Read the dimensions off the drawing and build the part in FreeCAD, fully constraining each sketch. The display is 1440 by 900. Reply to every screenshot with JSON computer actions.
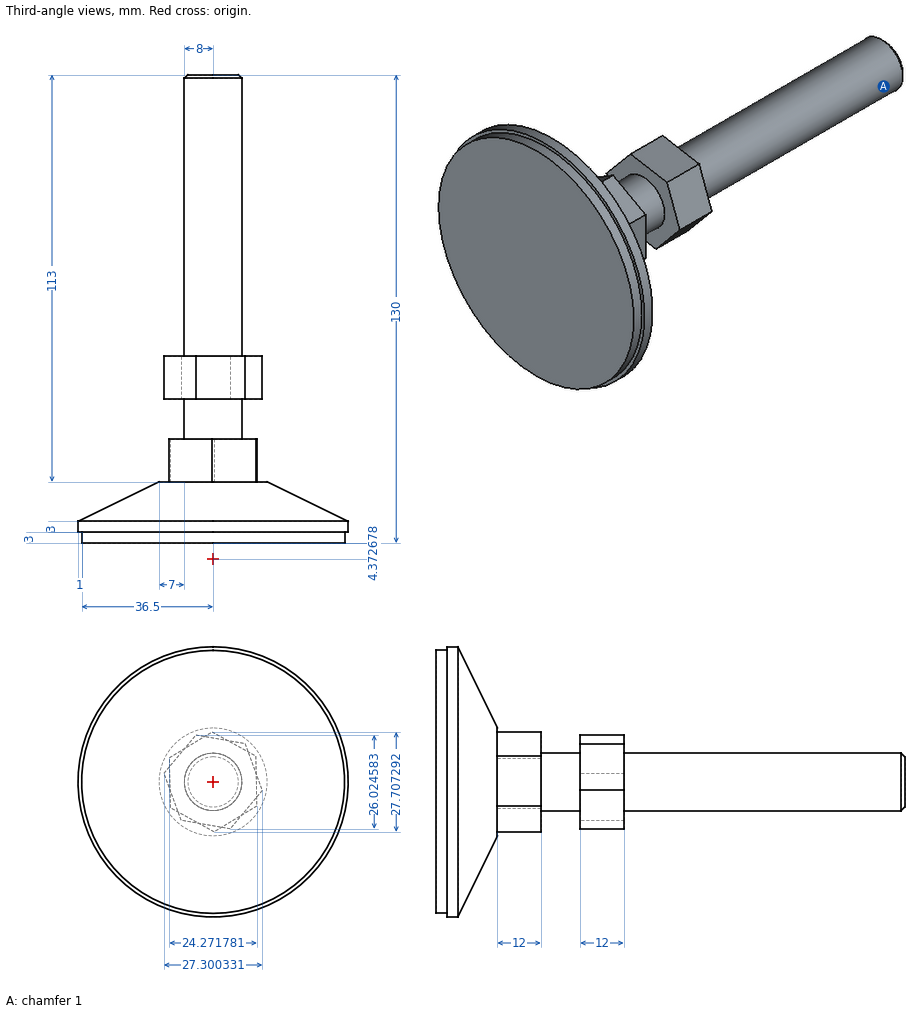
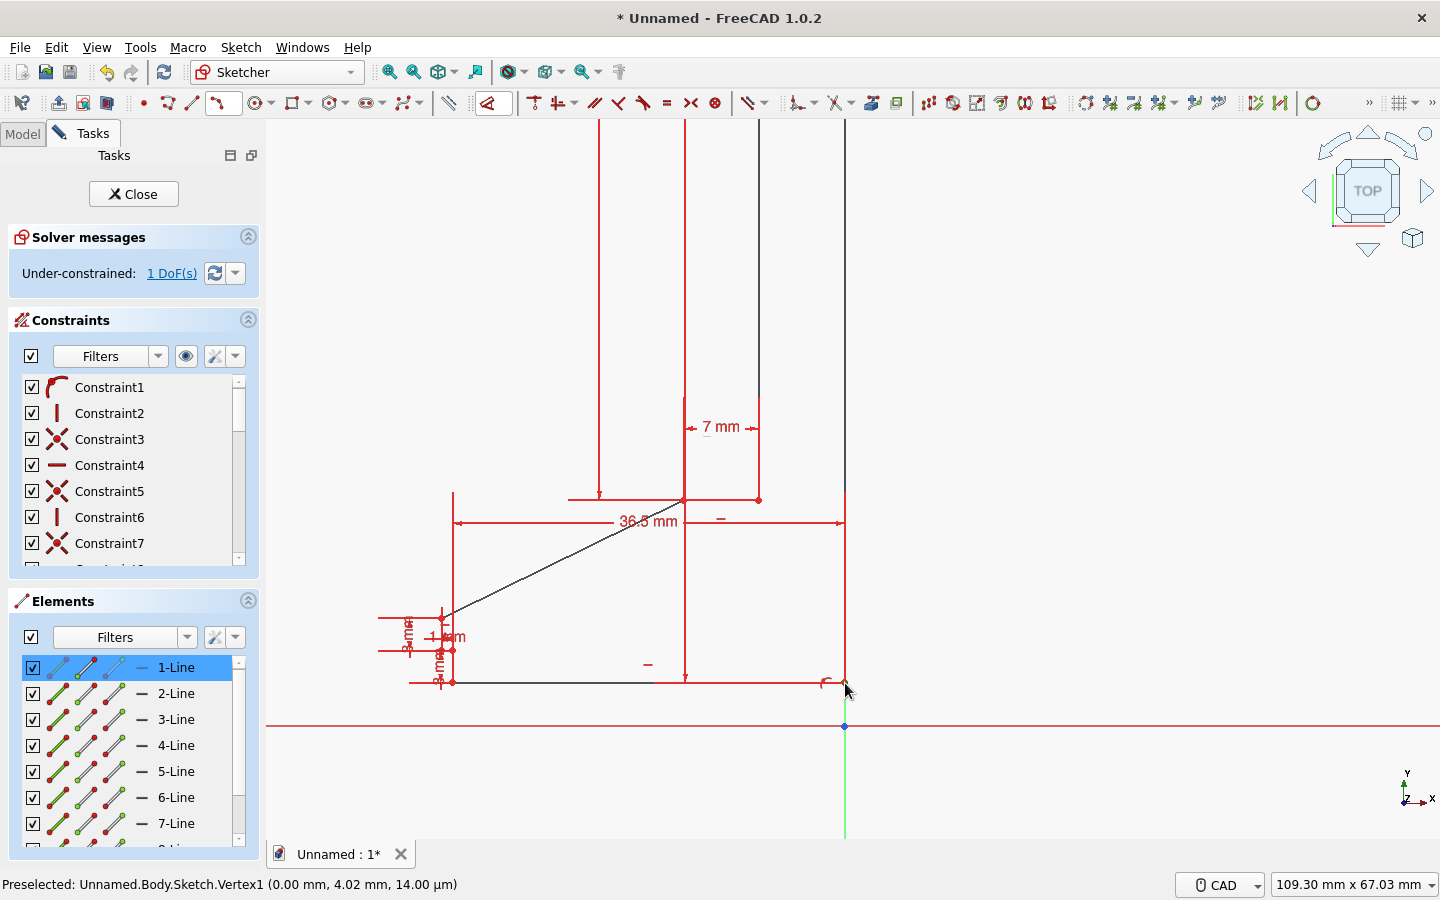
{"action": "key", "text": "i"}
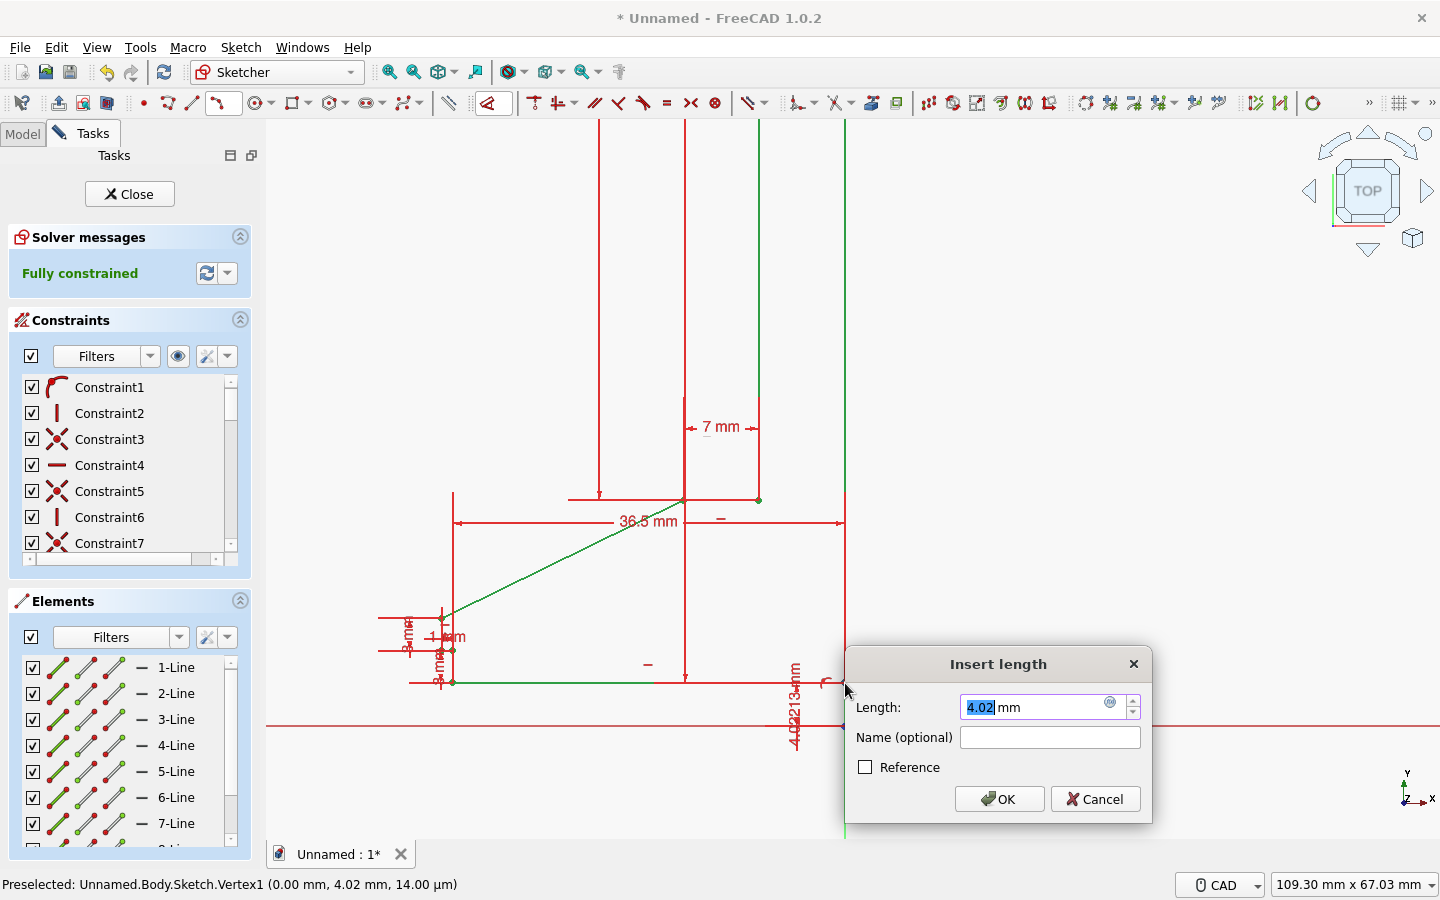
{"action": "type", "text": "4.372678"}
{"action": "key", "text": "Return"}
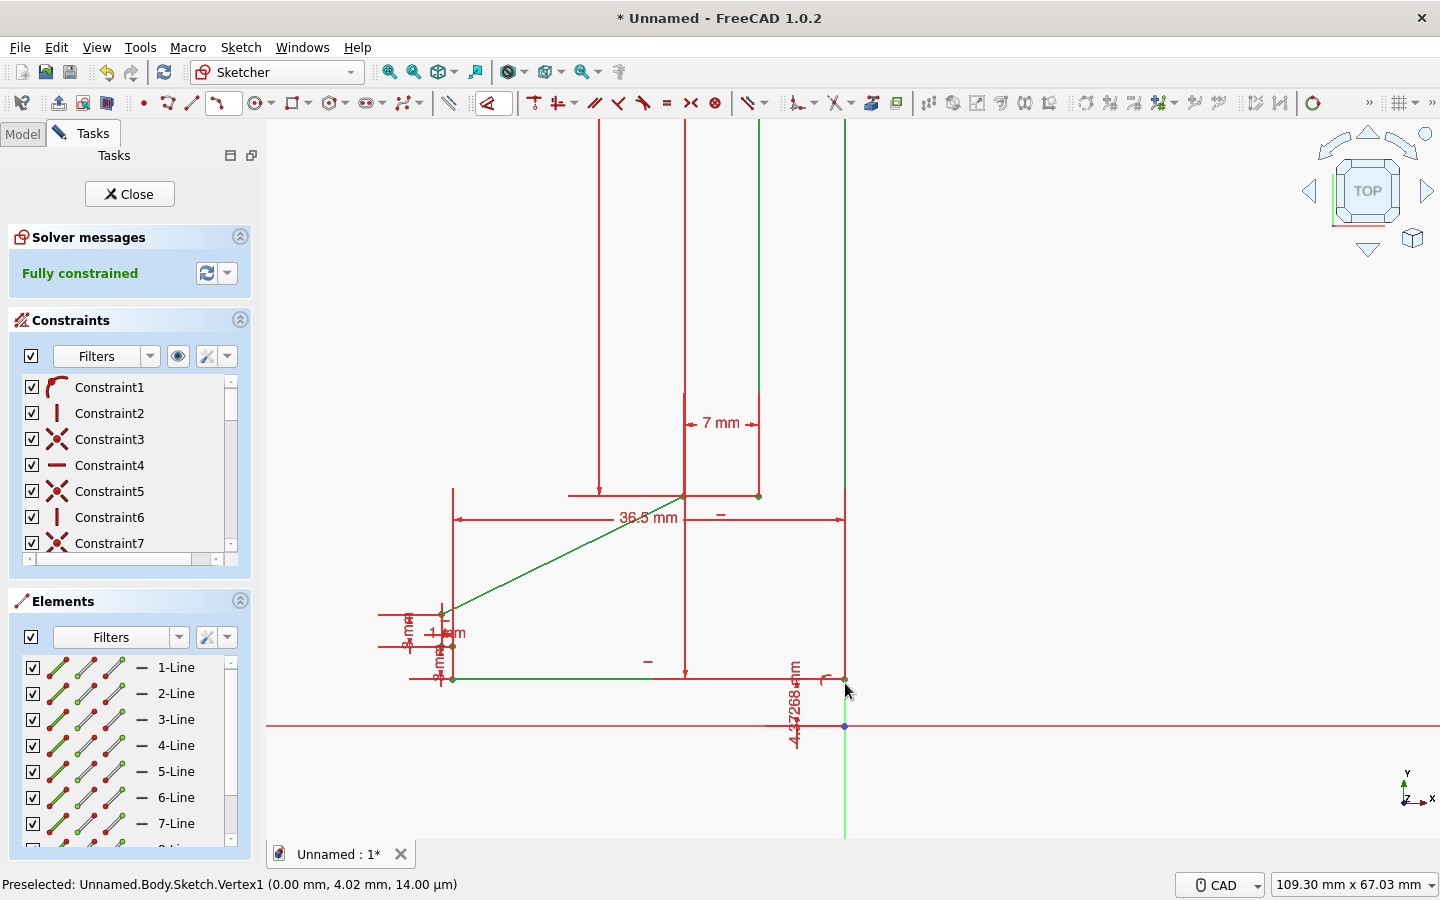
{"action": "left_click", "coordinate": [130, 194]}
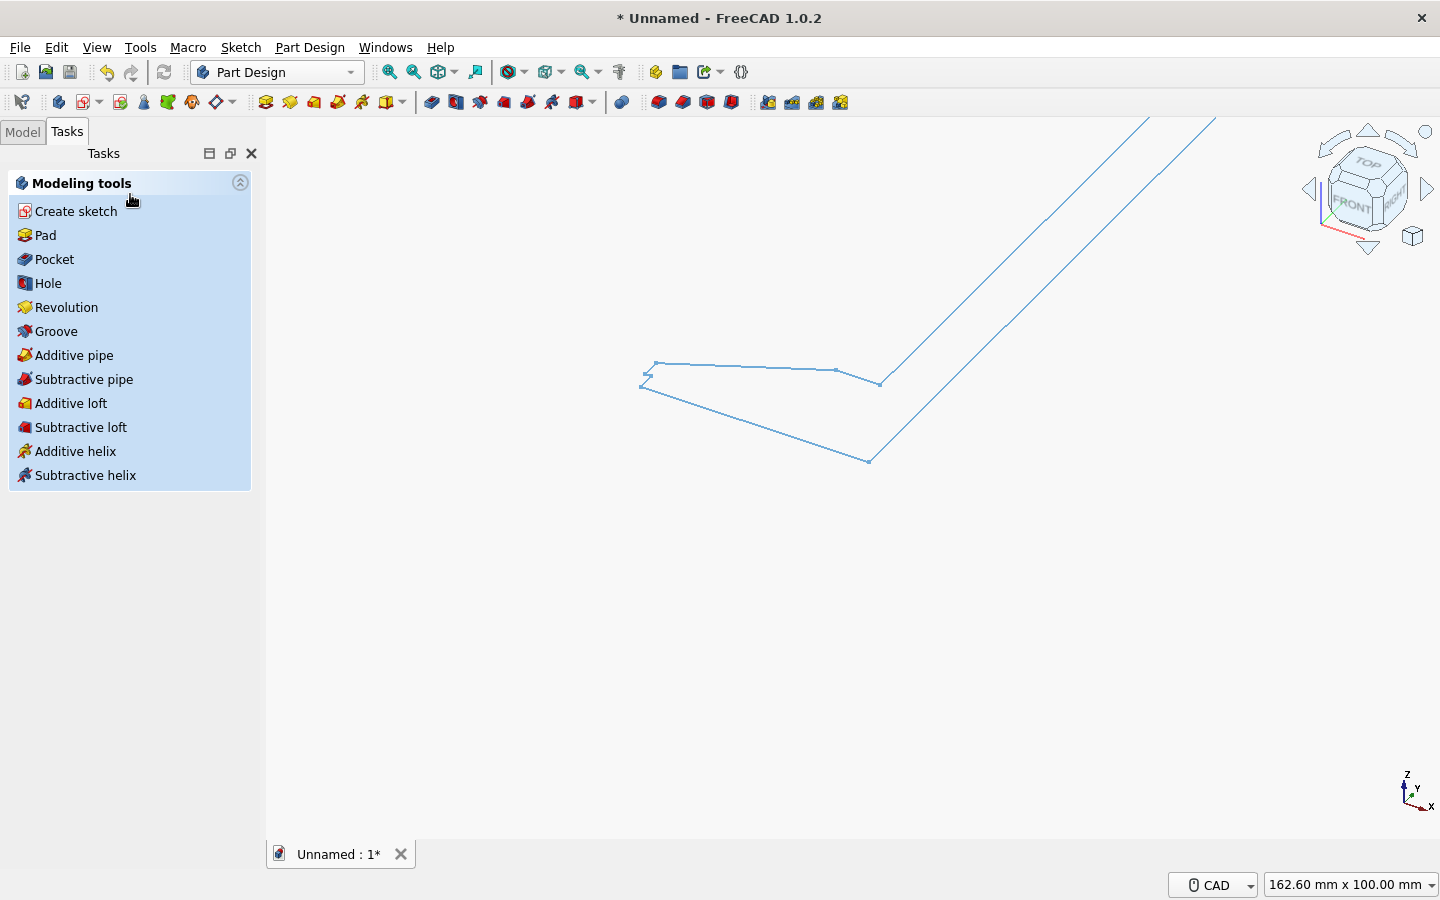
{"action": "left_click", "coordinate": [290, 102]}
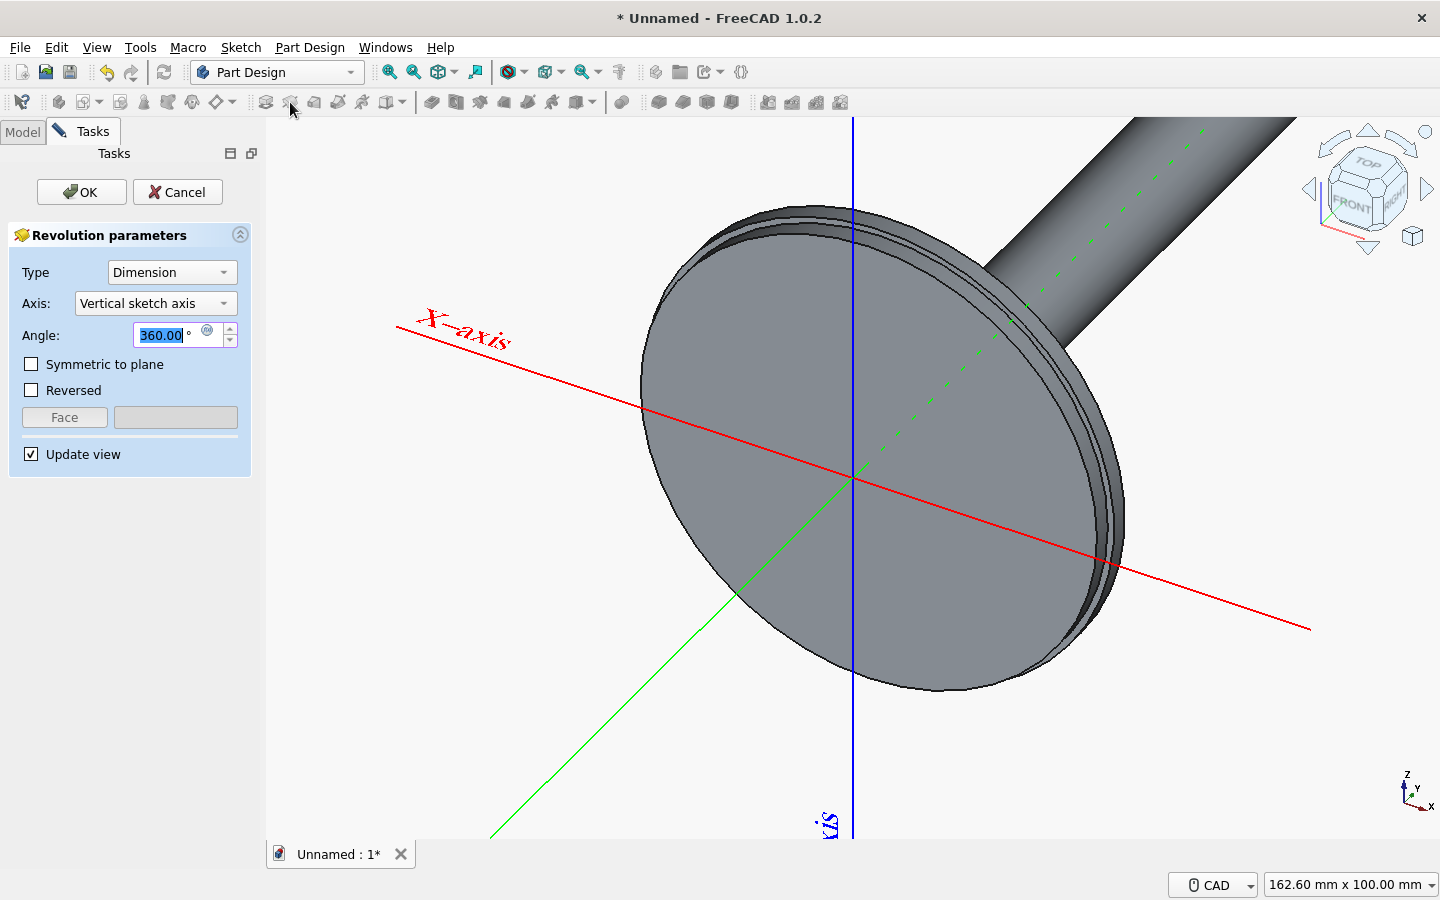
{"action": "left_click", "coordinate": [82, 192]}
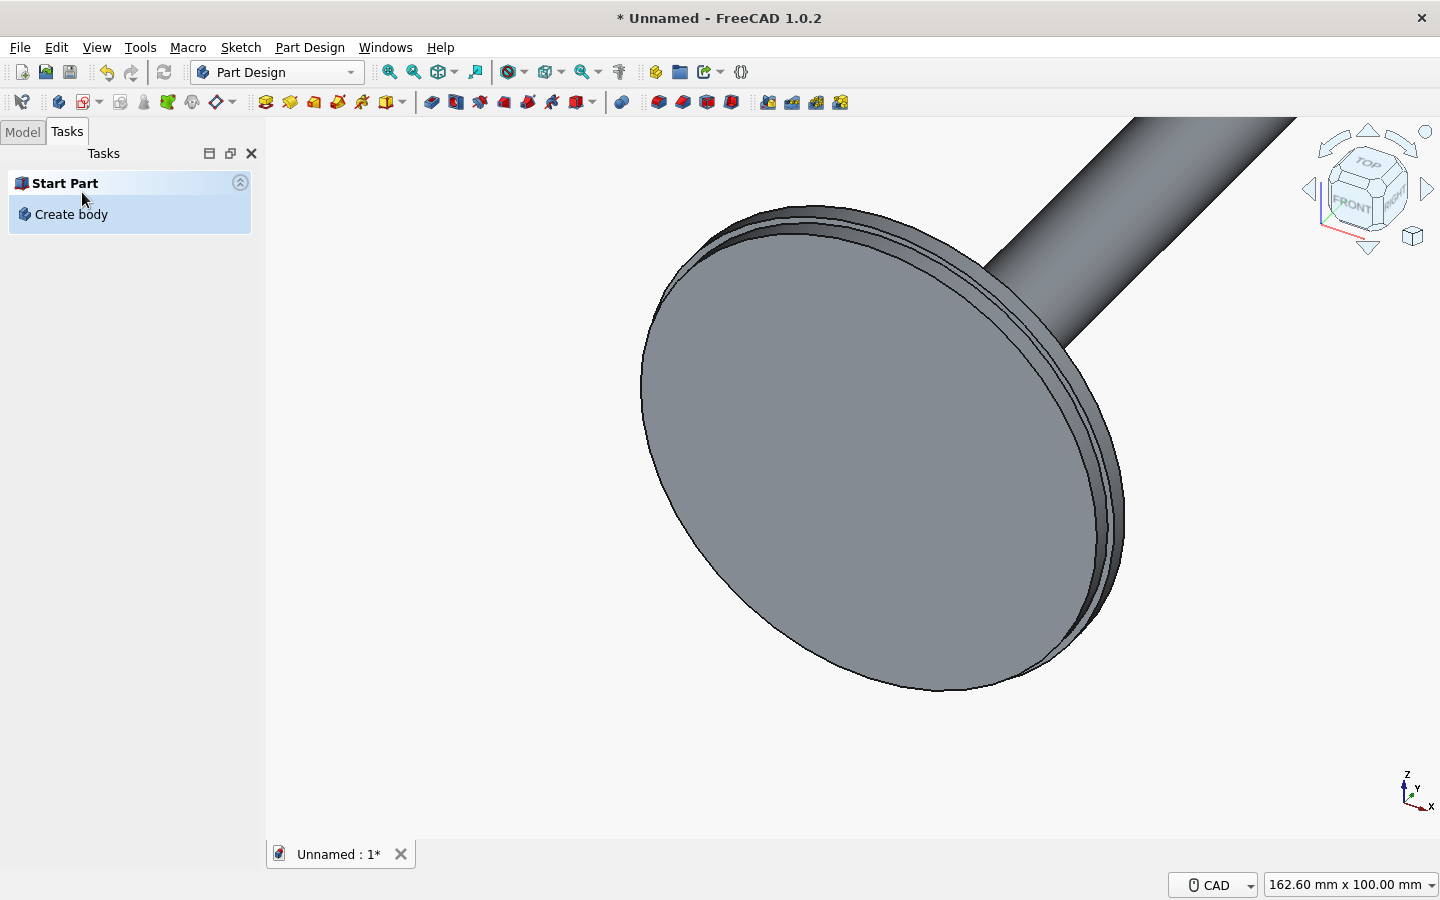
{"action": "left_click", "coordinate": [390, 72]}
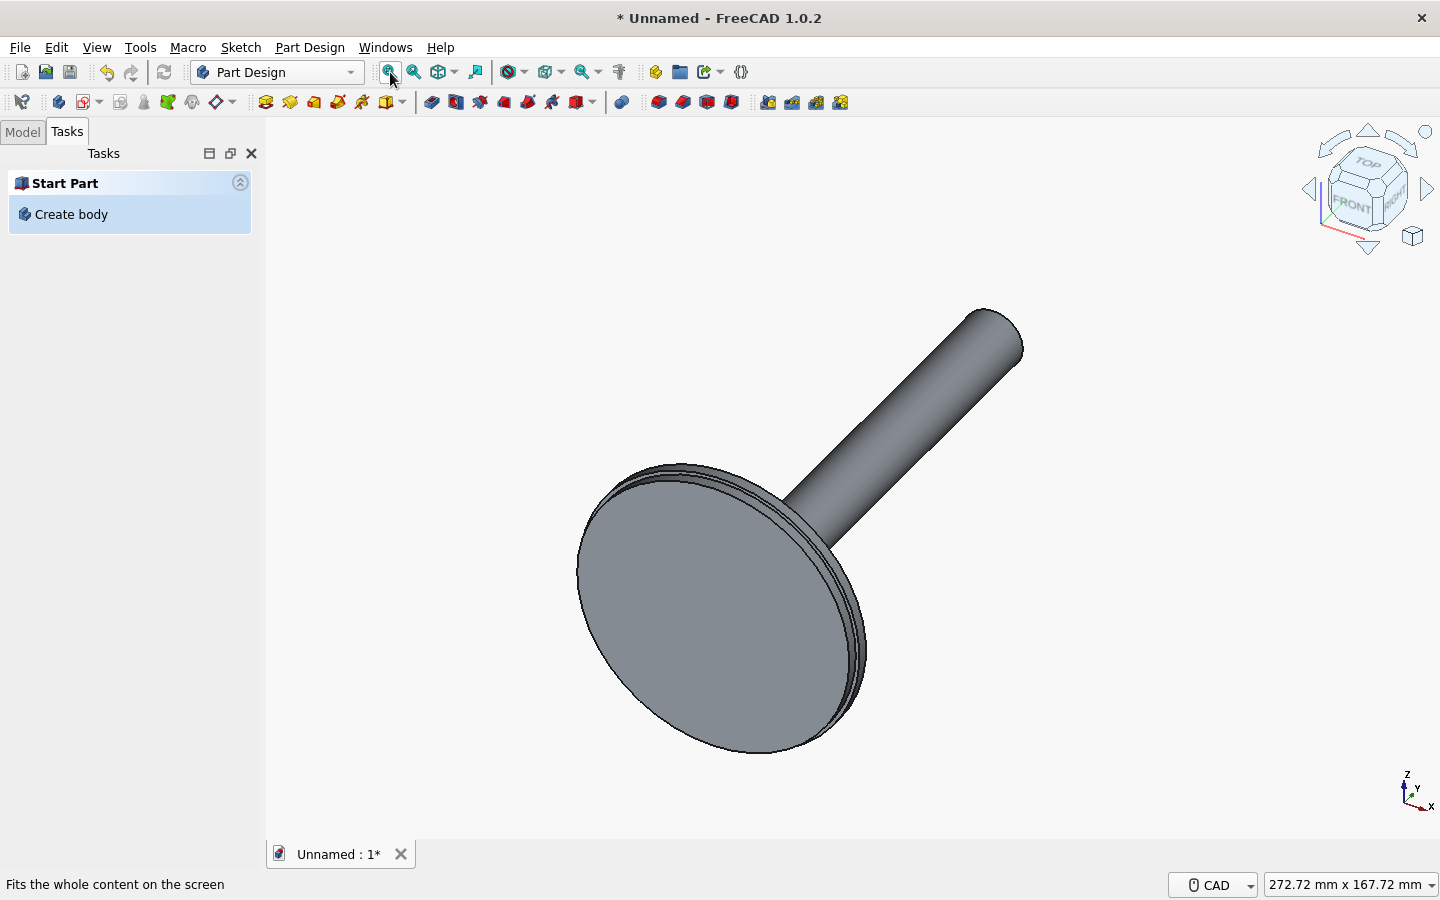
{"action": "key", "text": "4"}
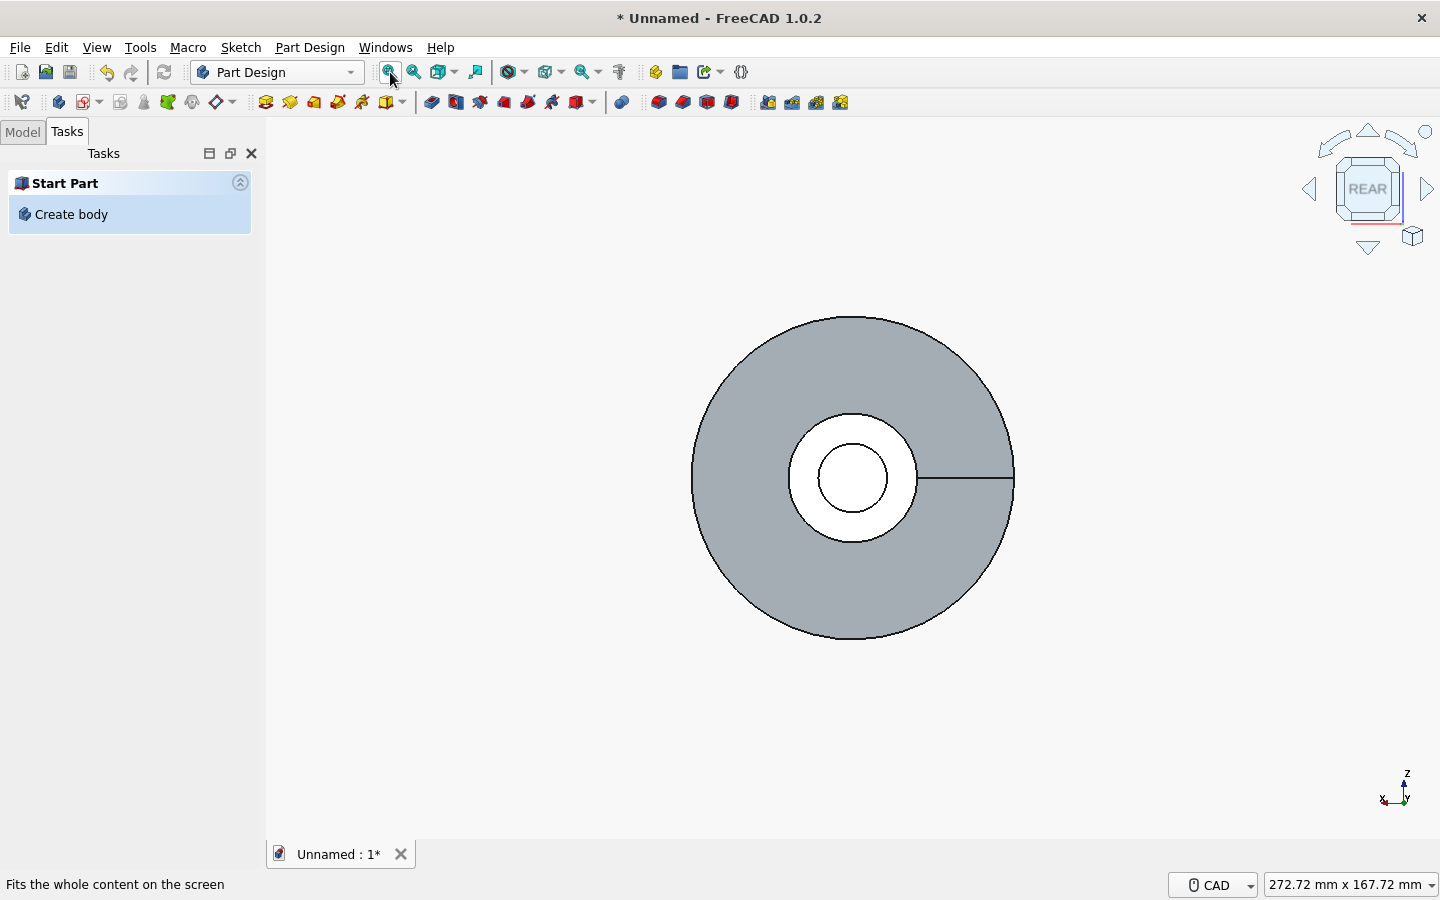
{"action": "left_click", "coordinate": [390, 72]}